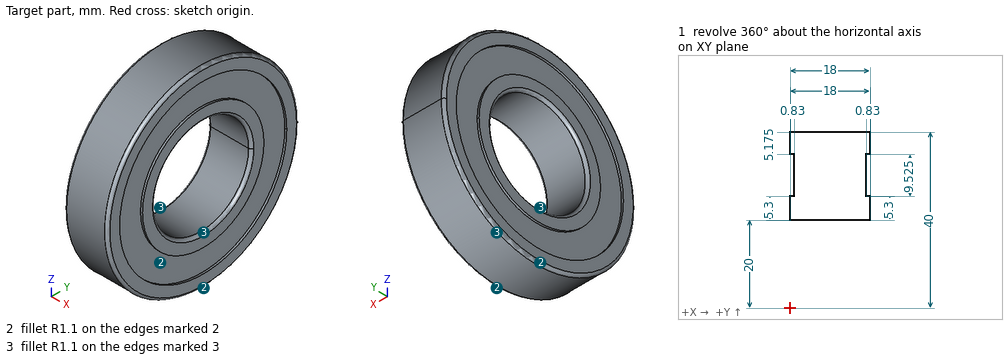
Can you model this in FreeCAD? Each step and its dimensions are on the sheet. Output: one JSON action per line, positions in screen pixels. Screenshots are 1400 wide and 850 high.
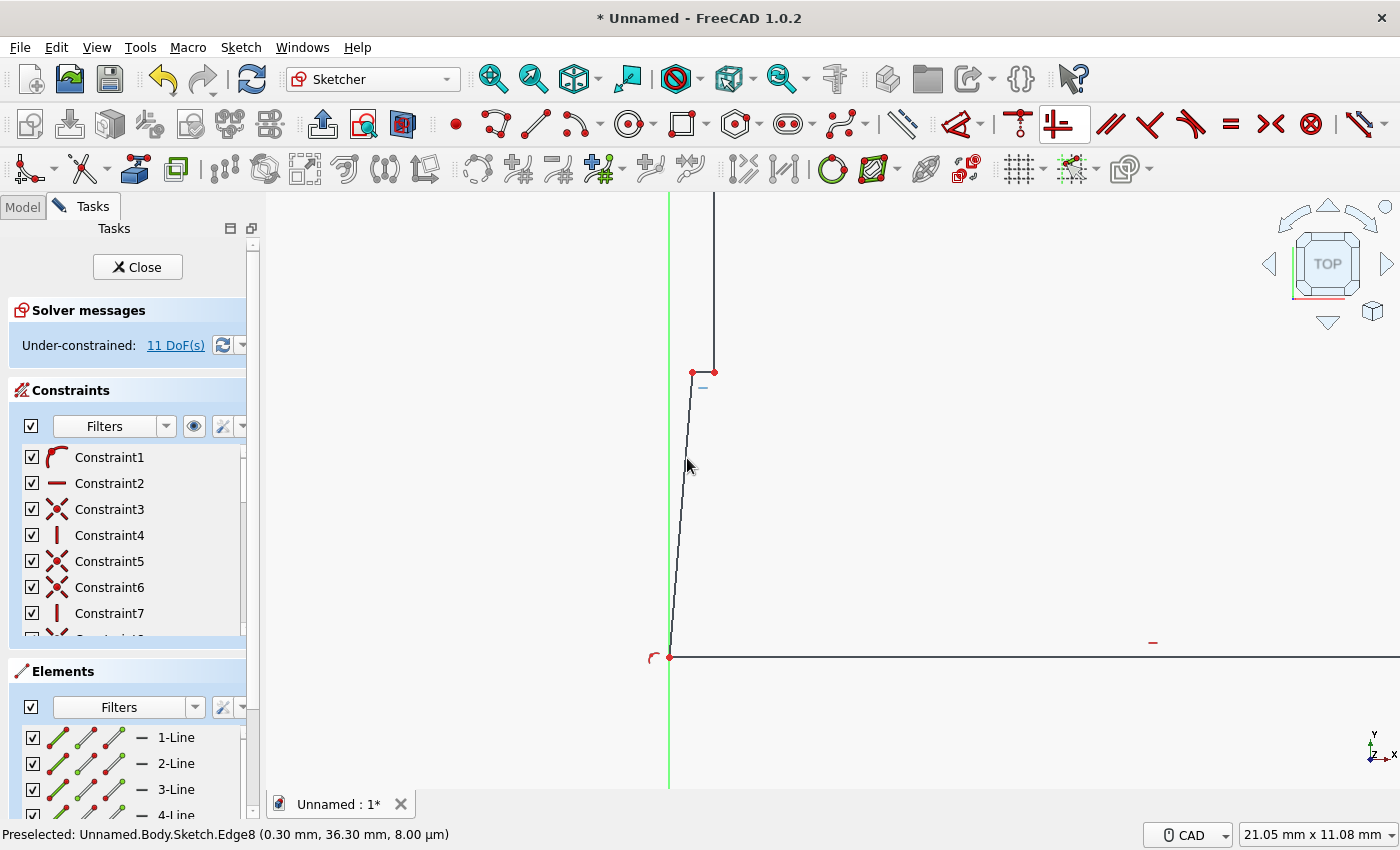
{"action": "left_click", "coordinate": [686, 458]}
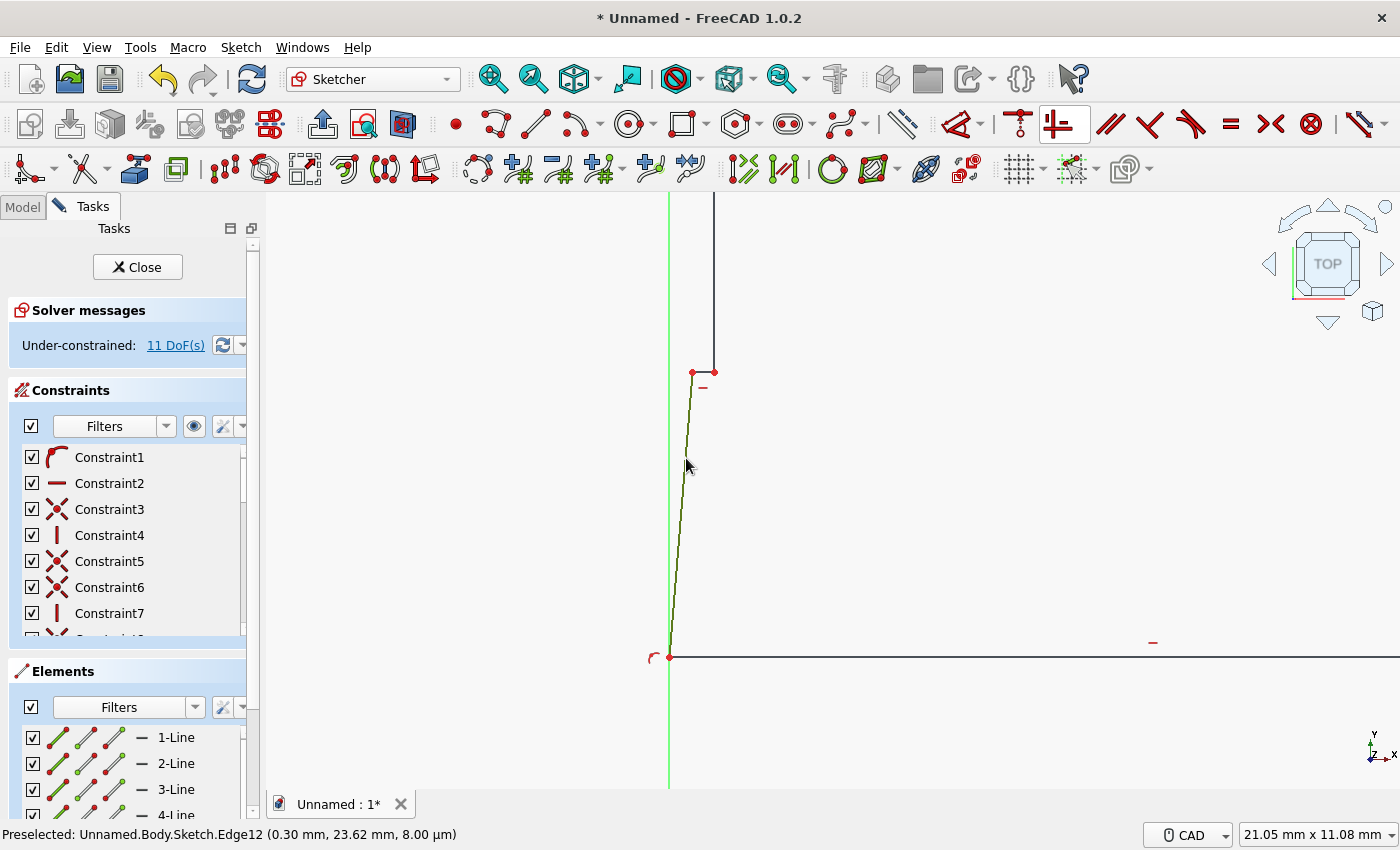
{"action": "key", "text": "v"}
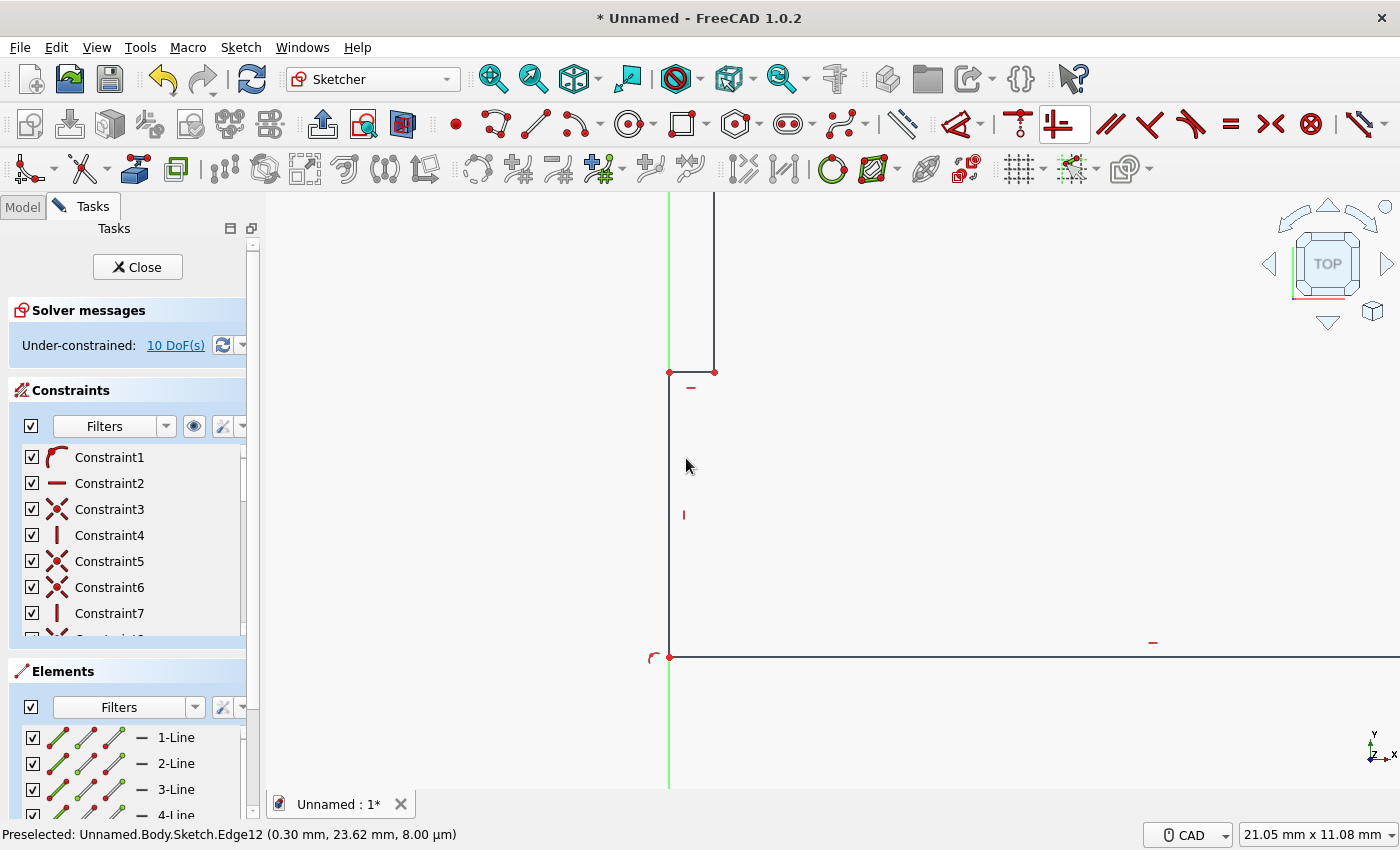
{"action": "left_click", "coordinate": [956, 124]}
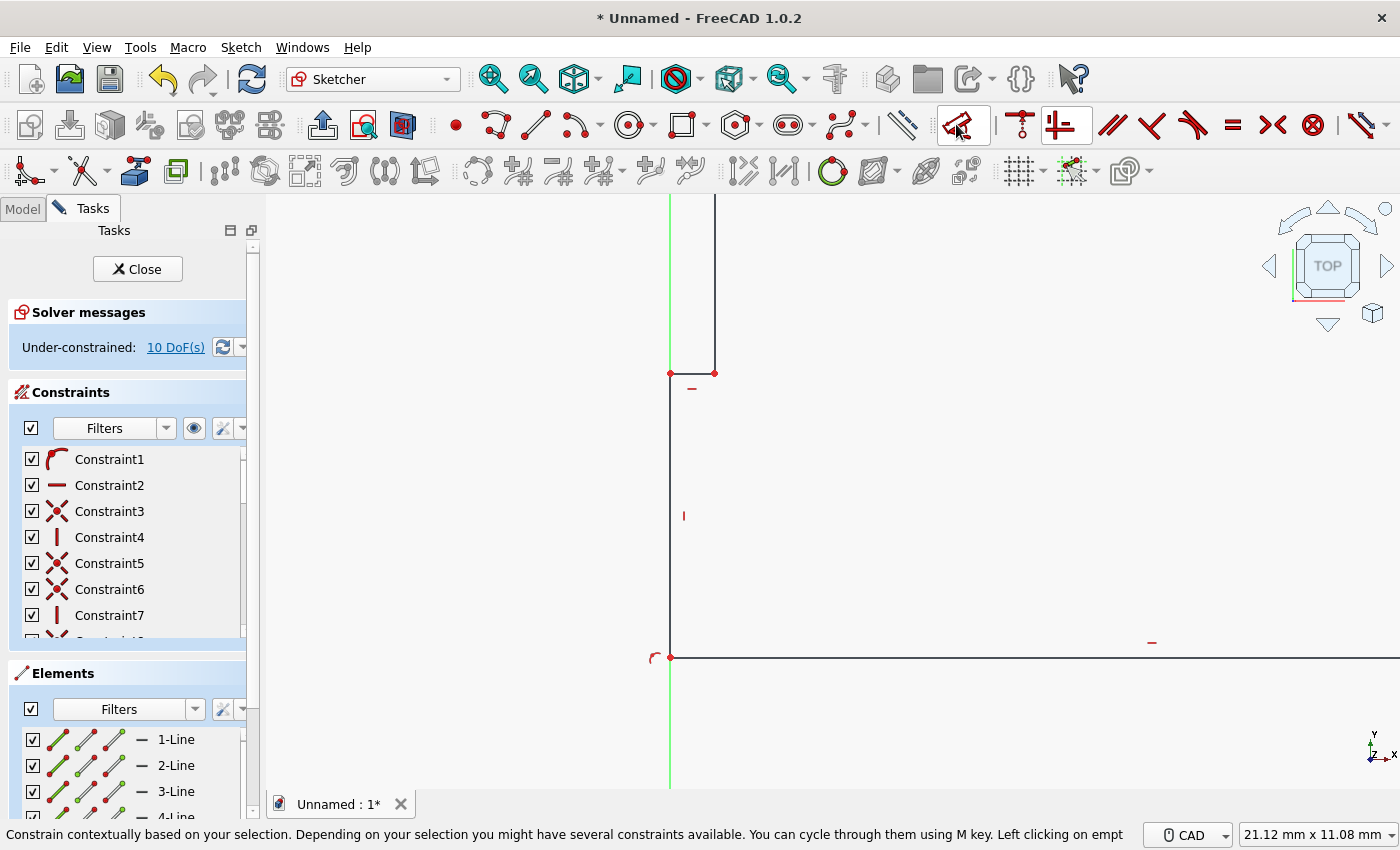
{"action": "scroll", "coordinate": [688, 459], "scroll_direction": "down", "scroll_amount": 9}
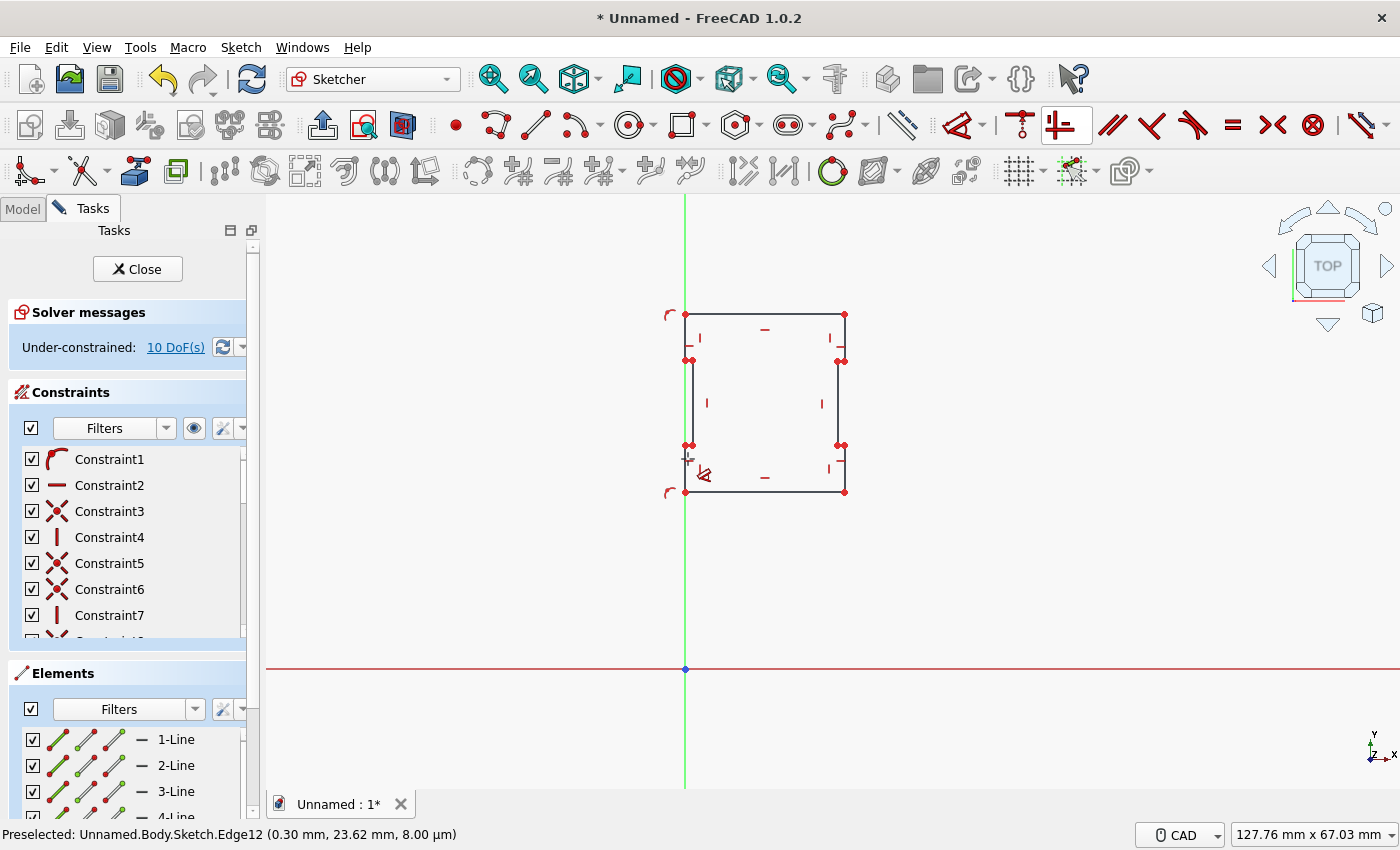
{"action": "left_click", "coordinate": [733, 492]}
{"action": "left_click", "coordinate": [765, 526]}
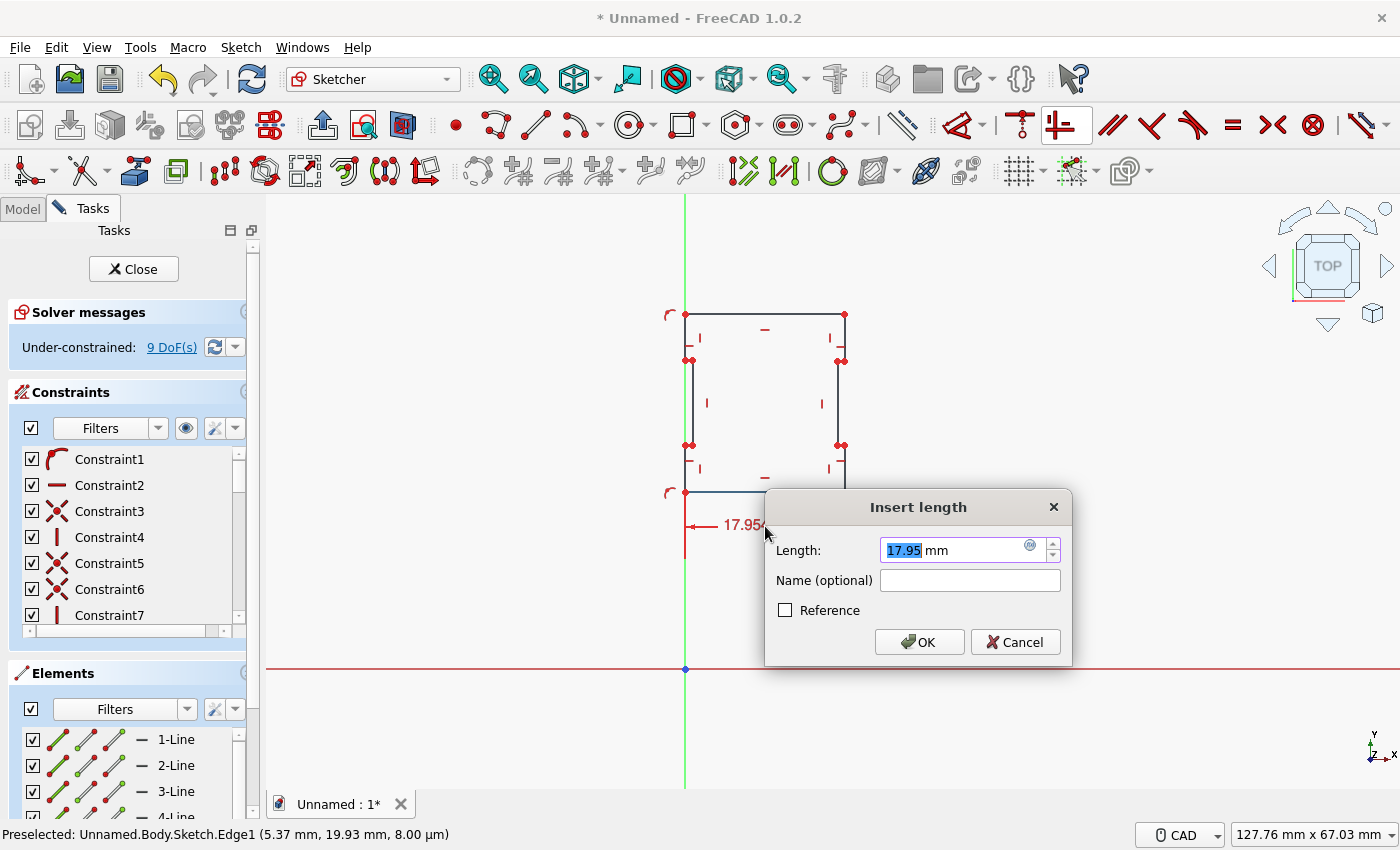
{"action": "type", "text": "18"}
{"action": "key", "text": "Return"}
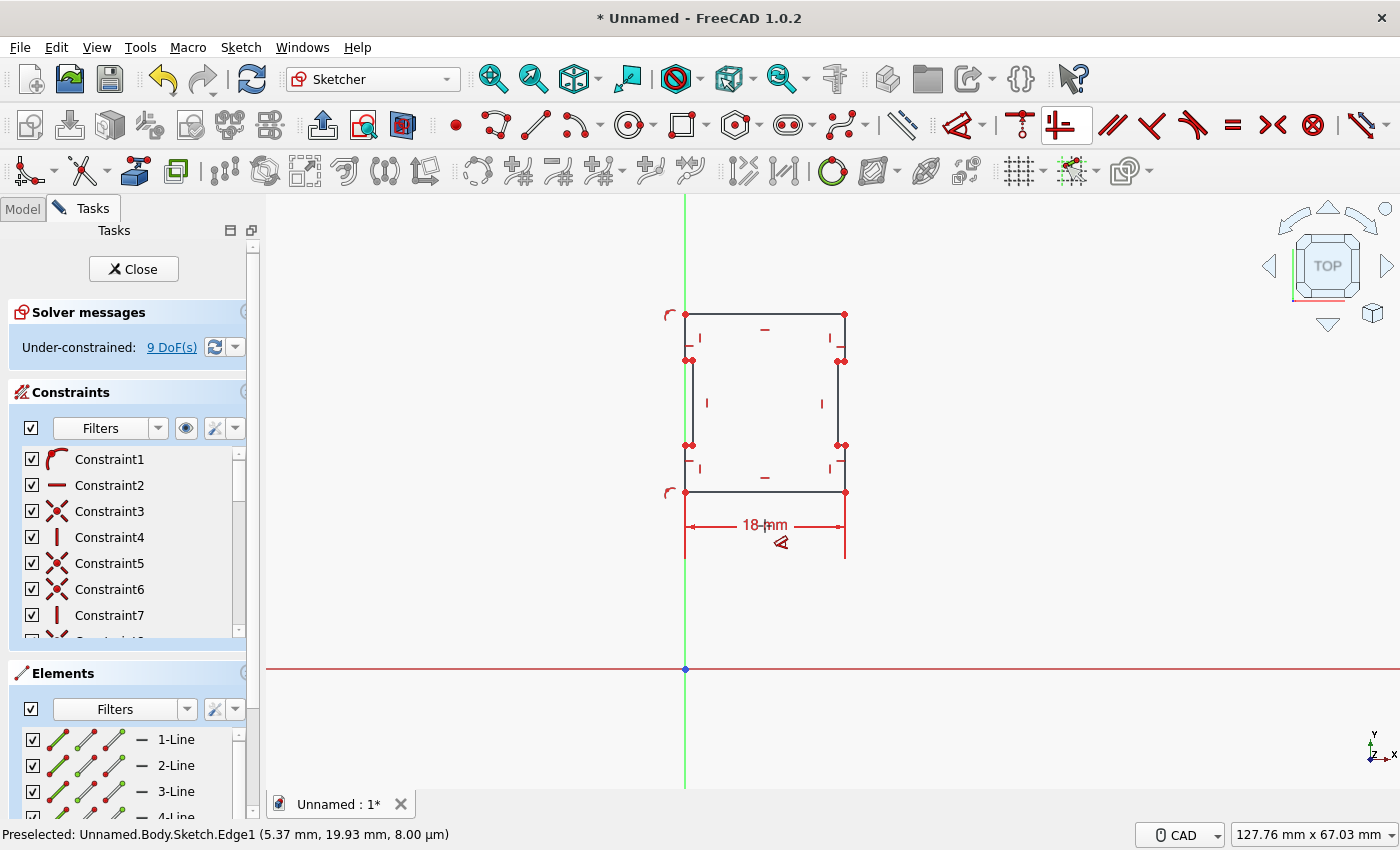
{"action": "left_click", "coordinate": [797, 314]}
{"action": "left_click", "coordinate": [765, 280]}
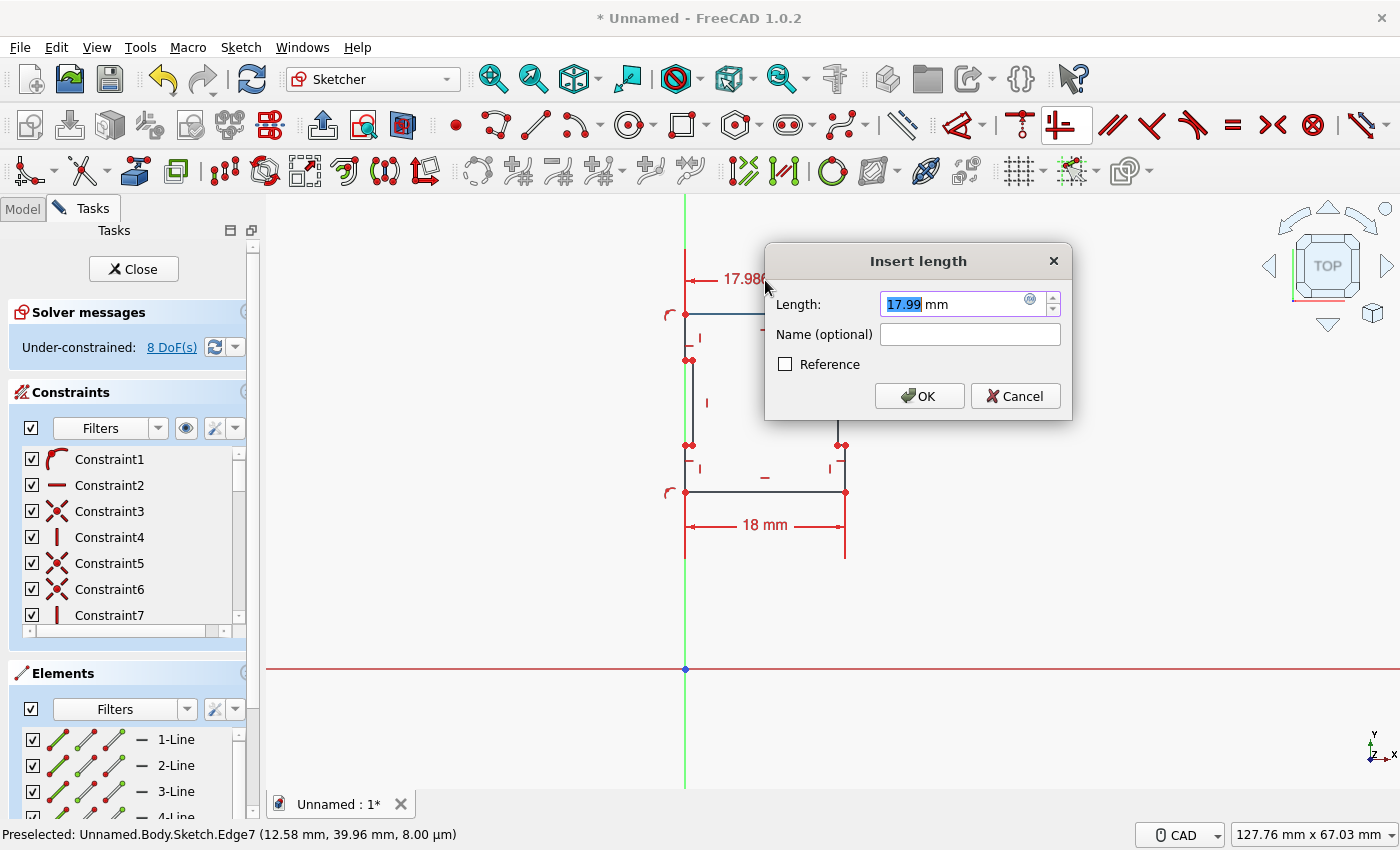
{"action": "type", "text": "18"}
{"action": "key", "text": "Return"}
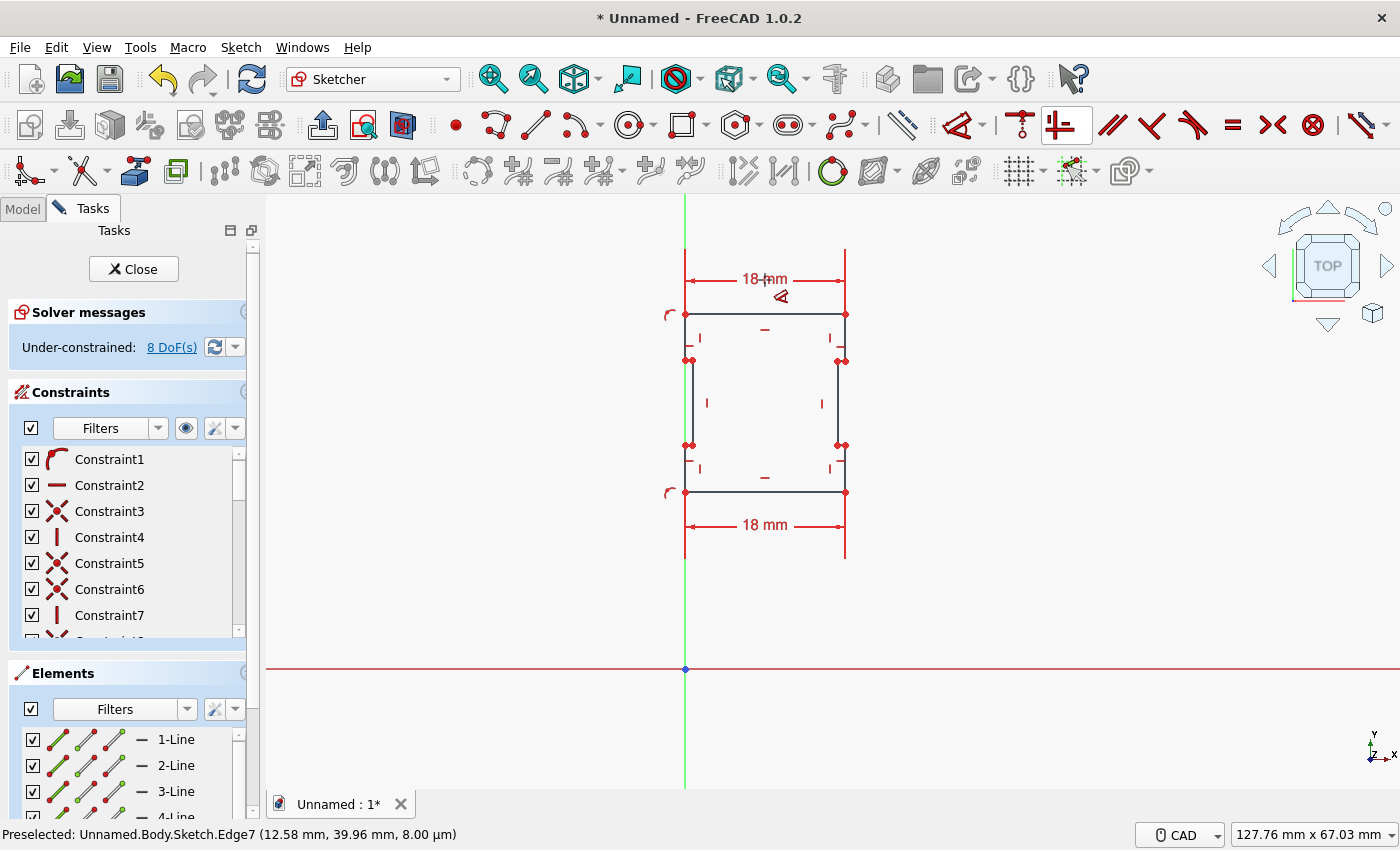
{"action": "left_click", "coordinate": [845, 478]}
{"action": "left_click", "coordinate": [879, 469]}